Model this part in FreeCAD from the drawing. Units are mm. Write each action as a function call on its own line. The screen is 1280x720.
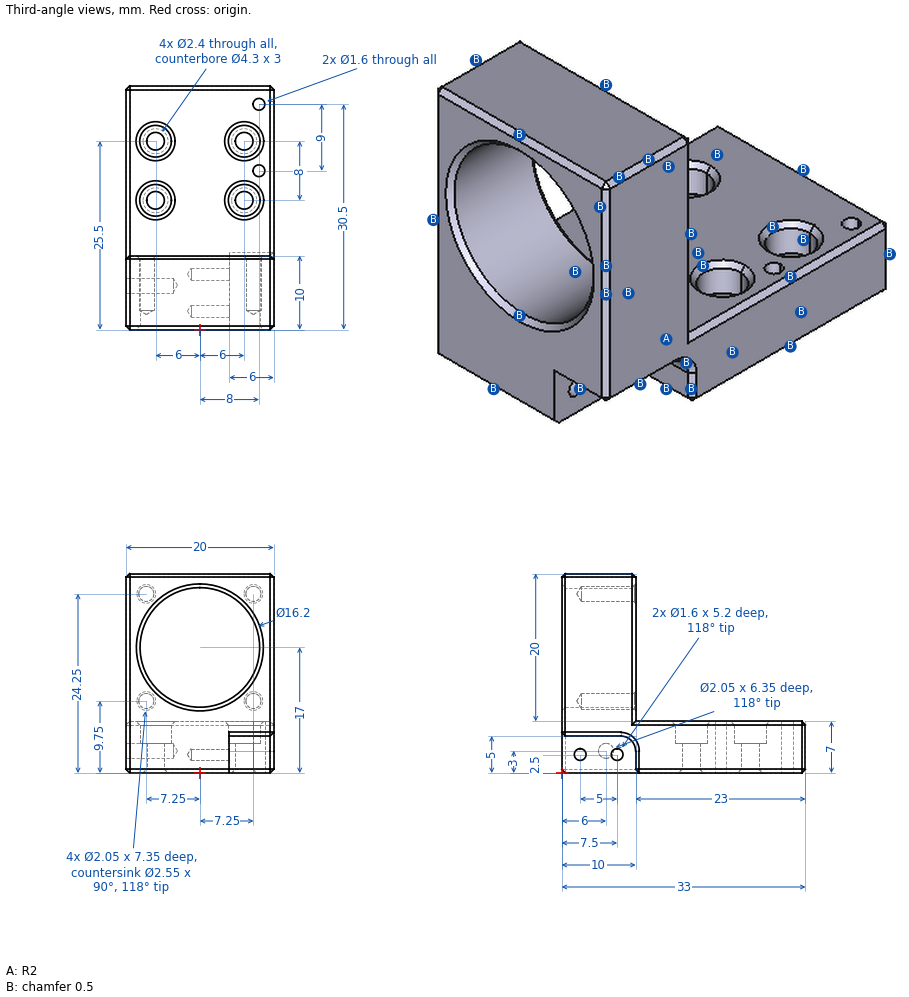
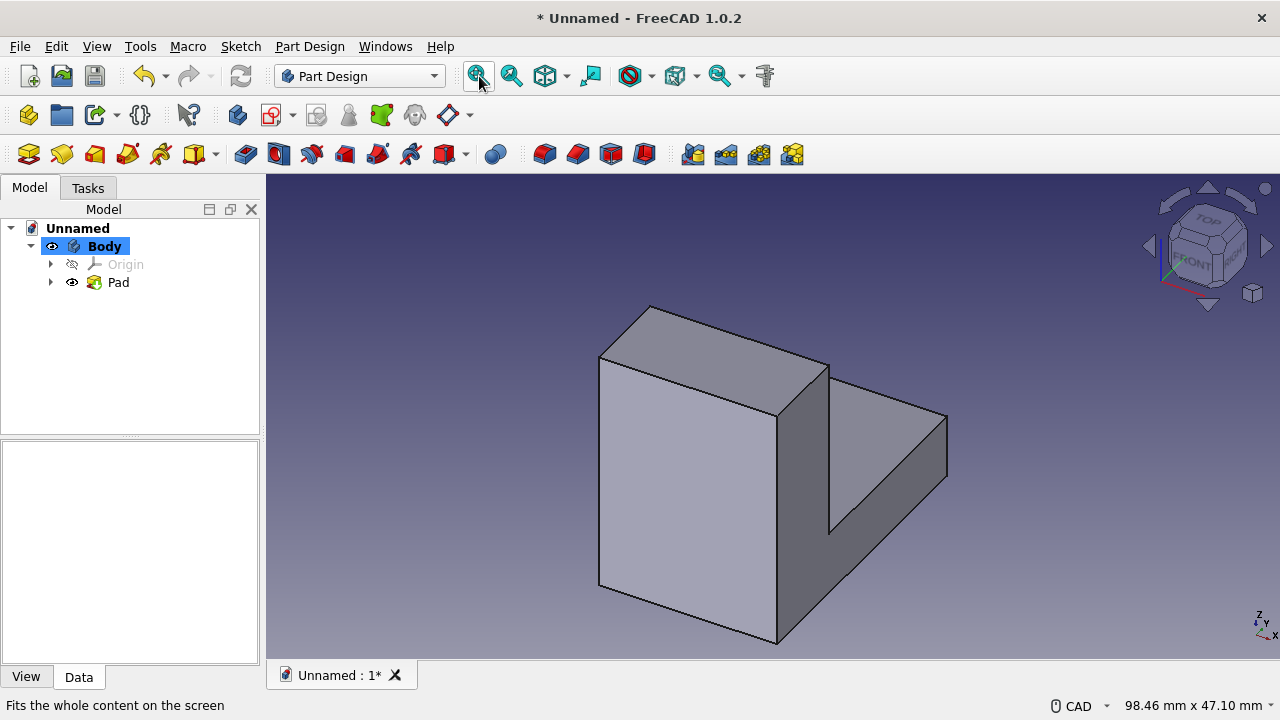
key(4)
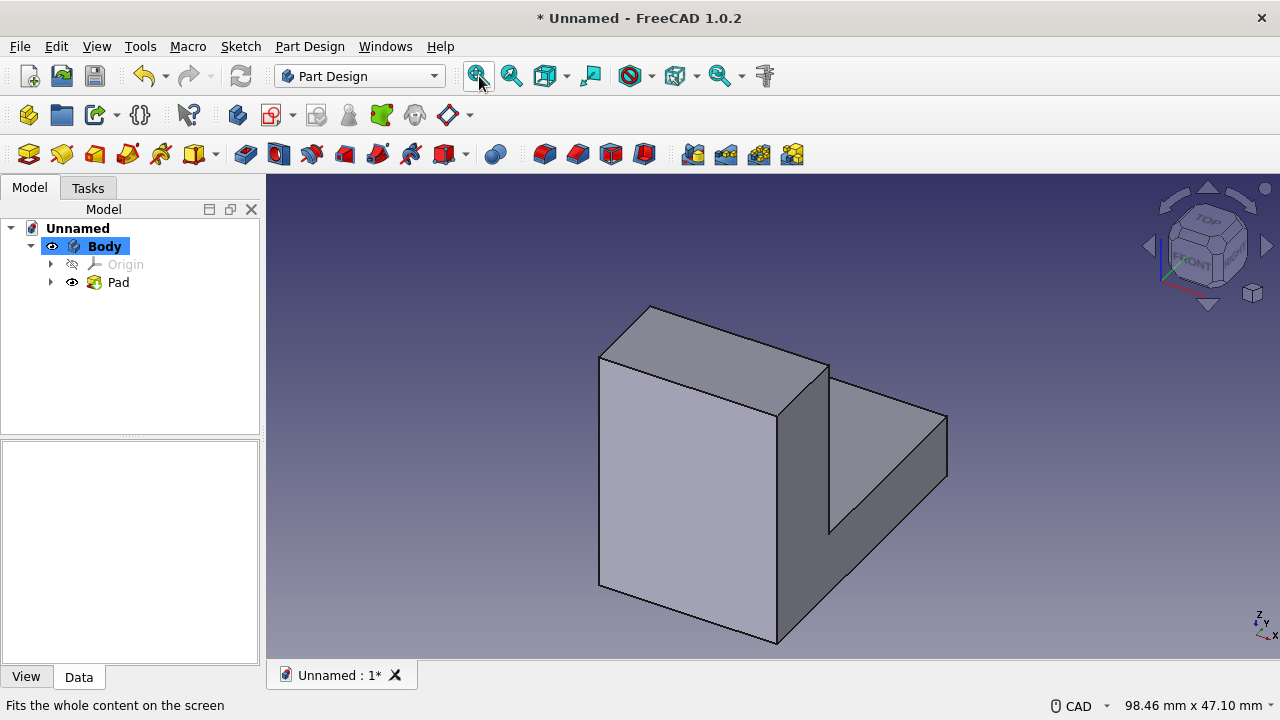
click(773, 379)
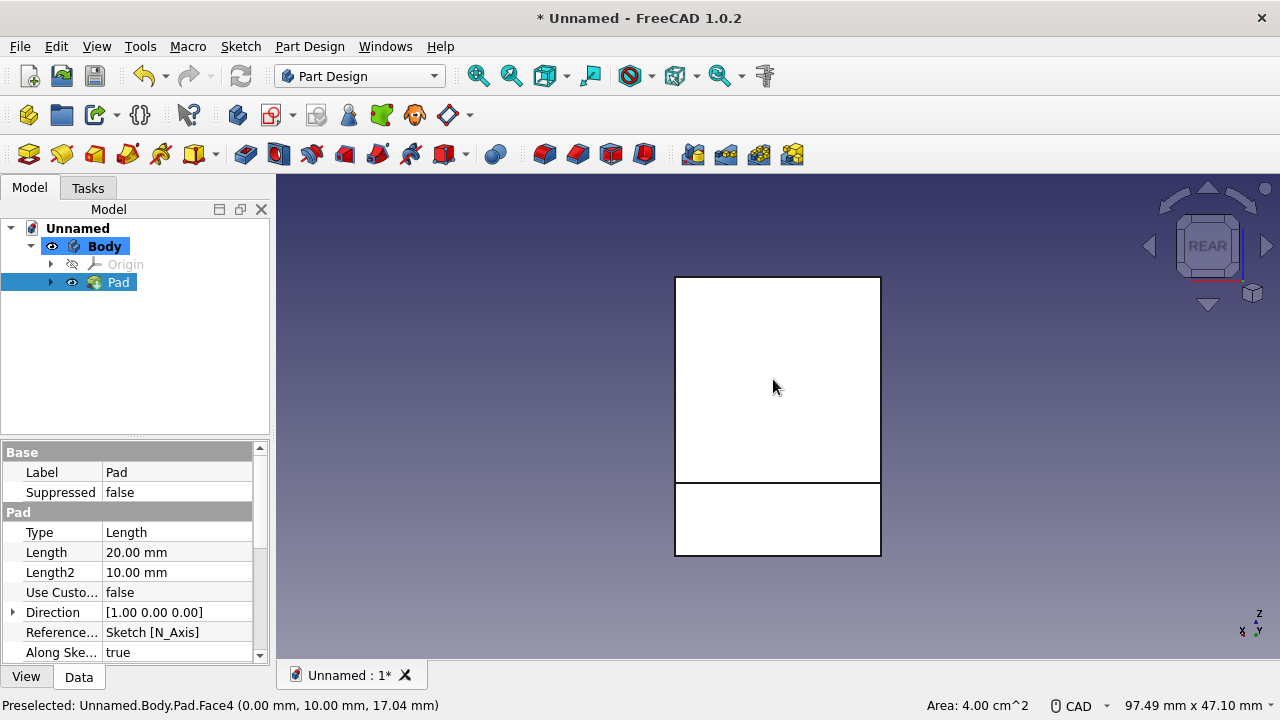
click(270, 116)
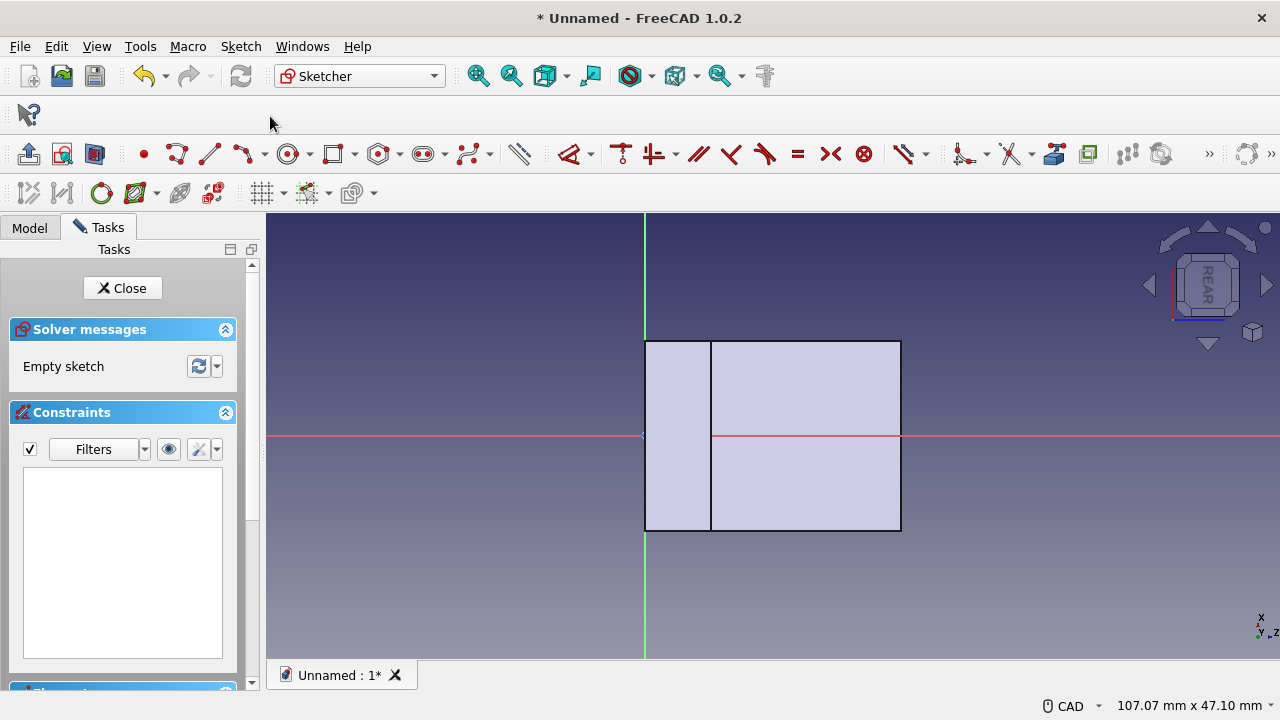
click(95, 154)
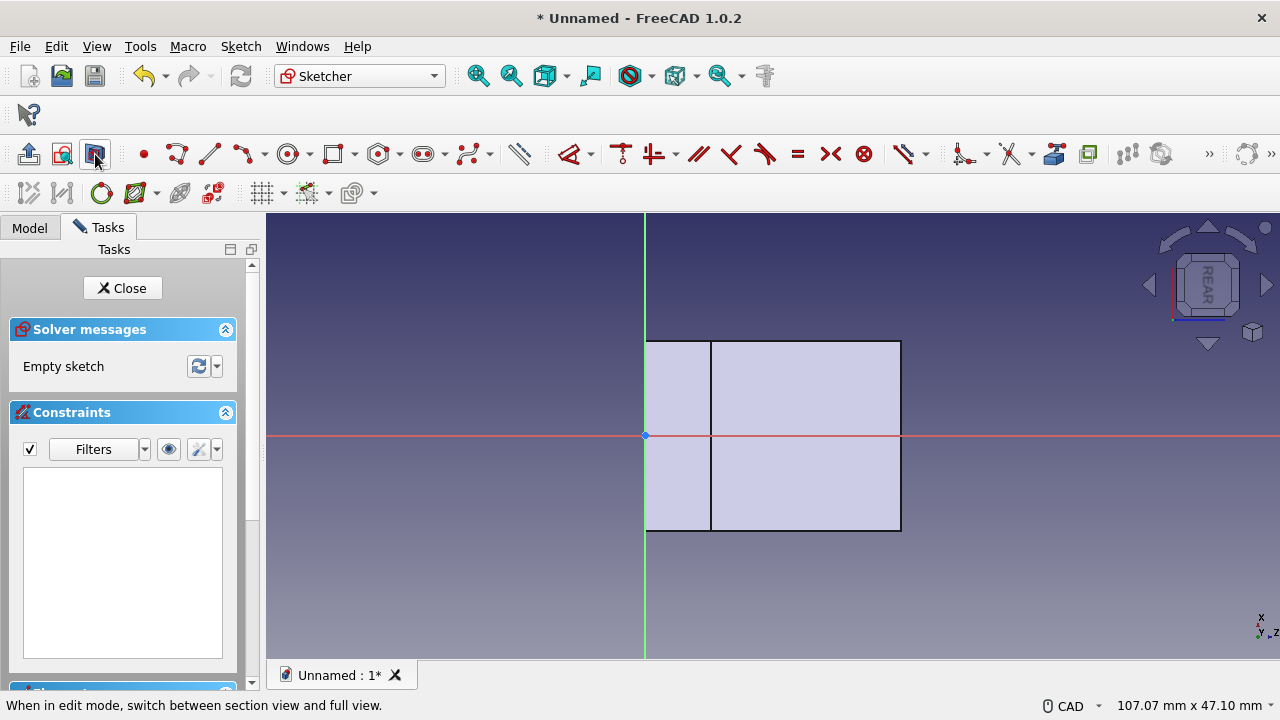
scroll(836, 436, up, 3)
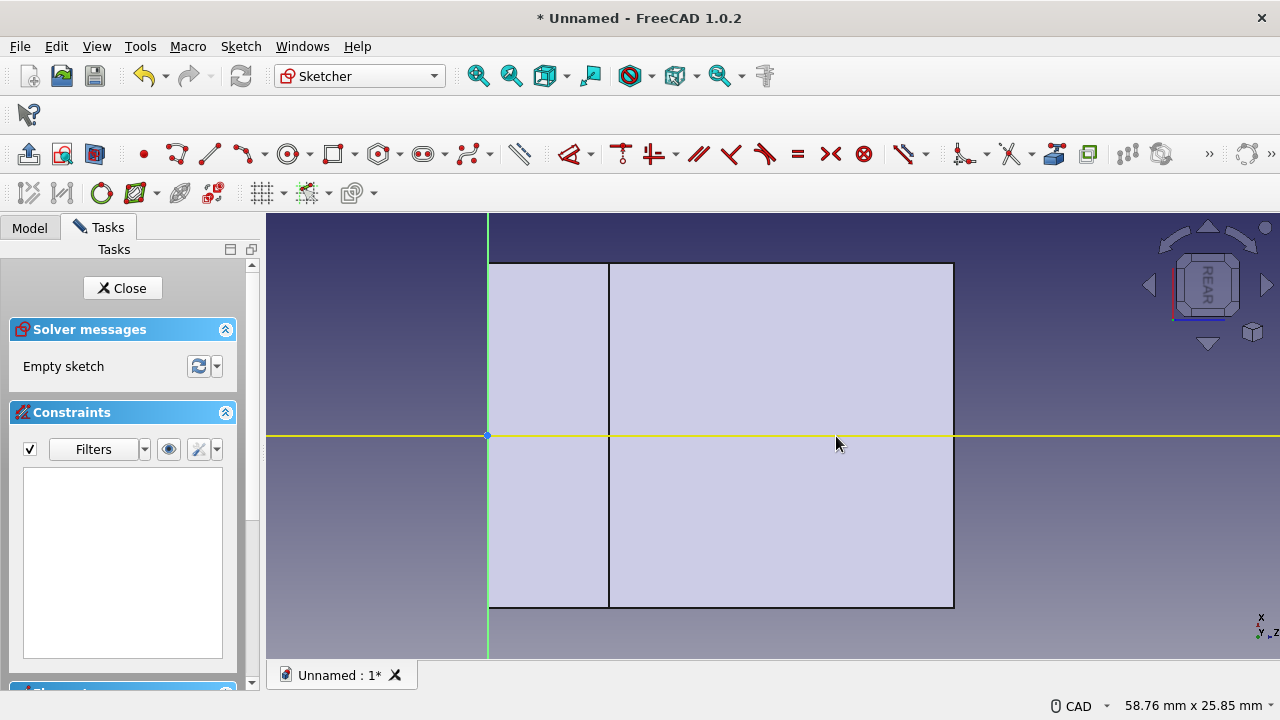
key(g)
key(c)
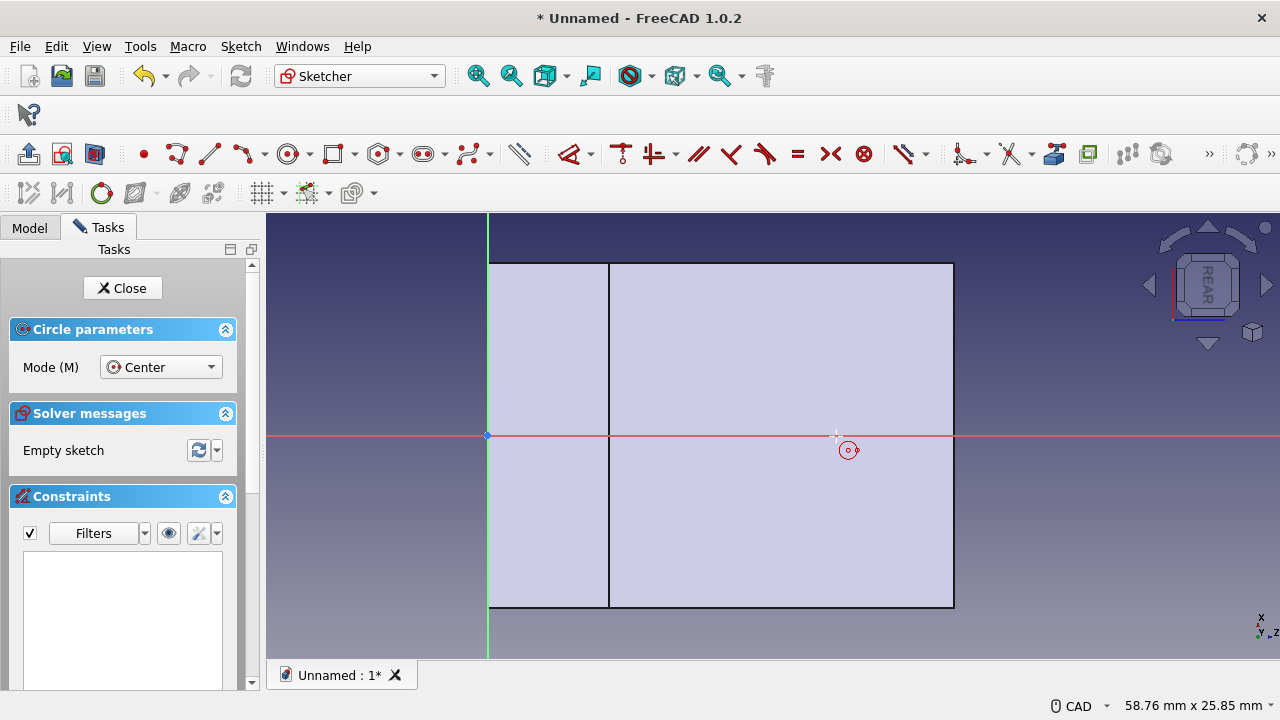
click(781, 436)
move(880, 337)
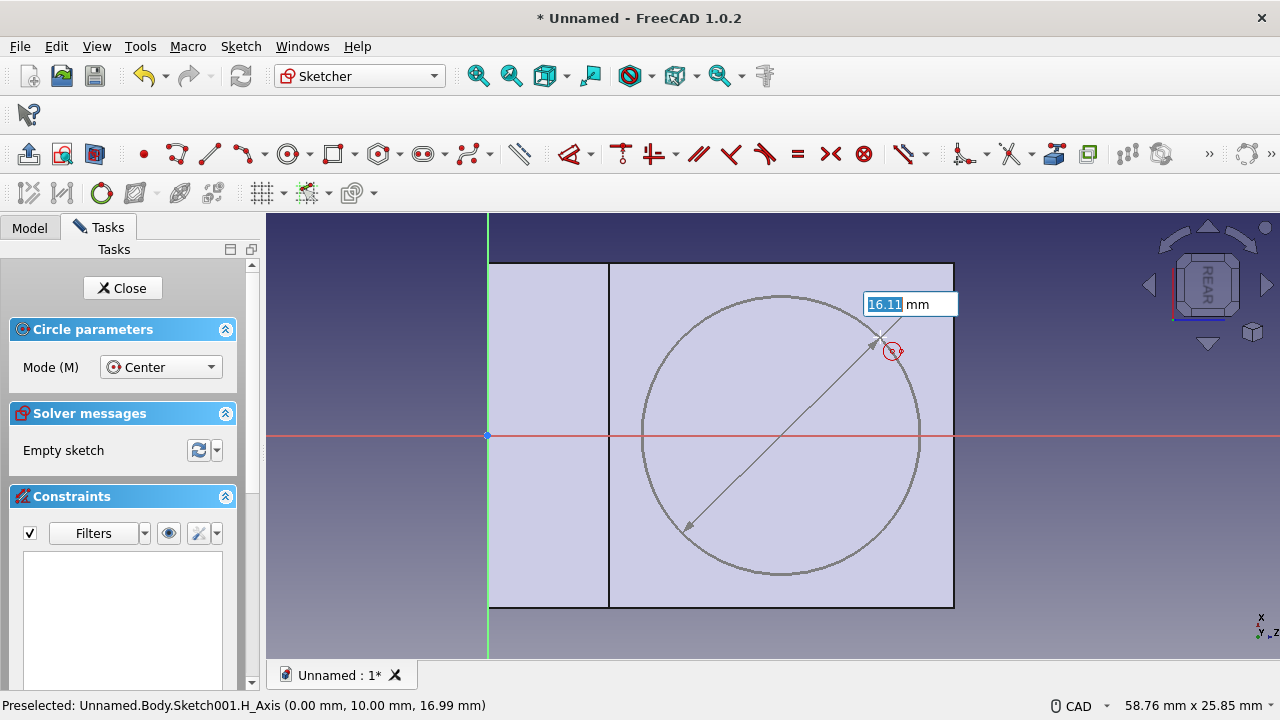
text(16.2)
key(Return)
key(Escape)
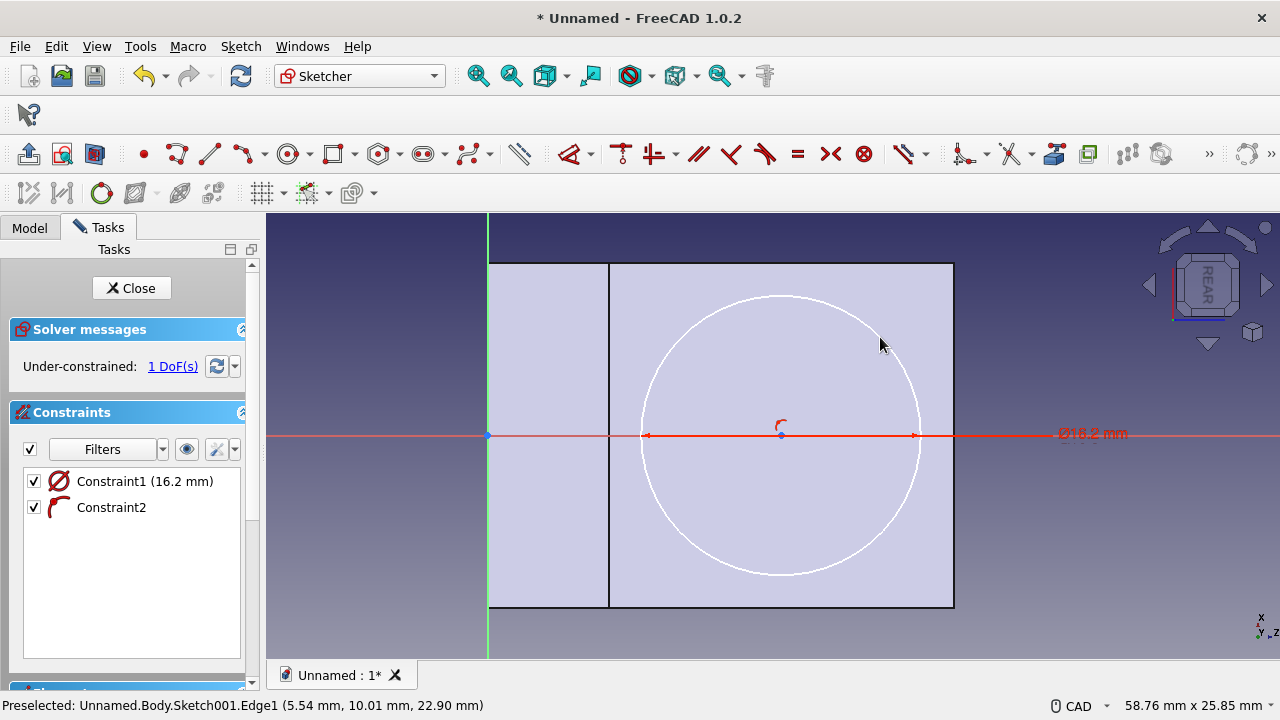
click(568, 154)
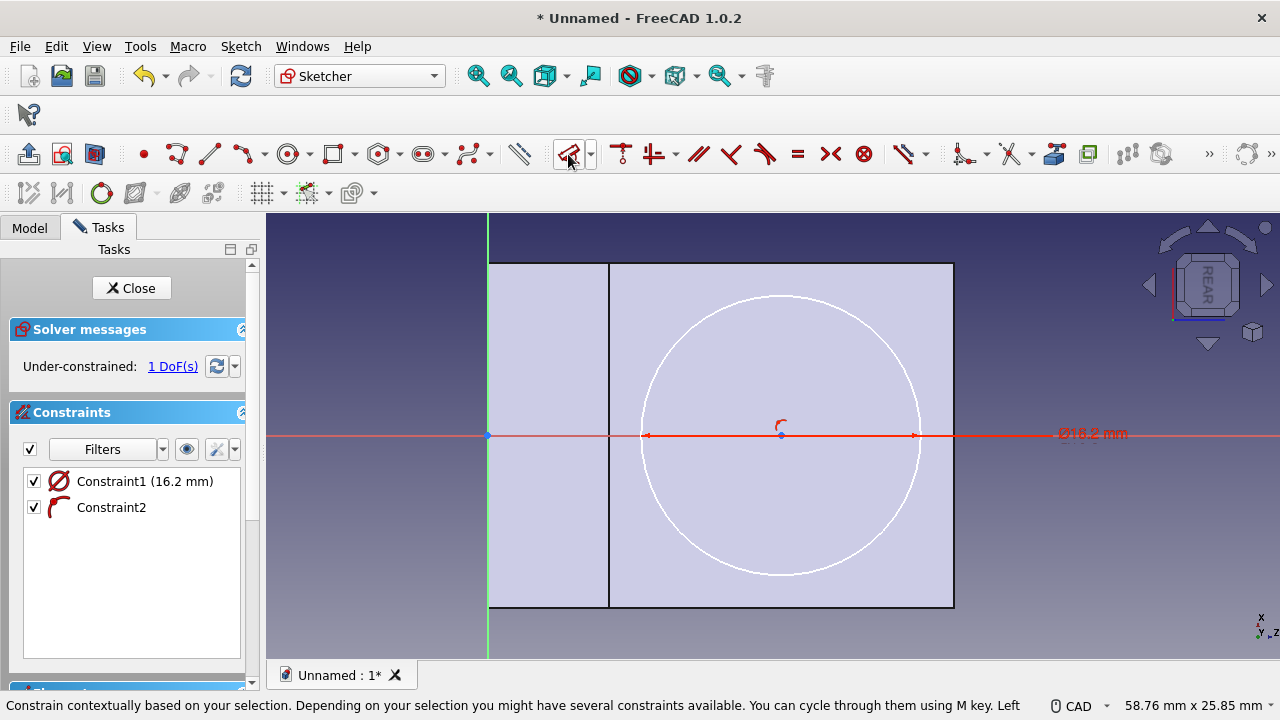
click(781, 436)
click(567, 470)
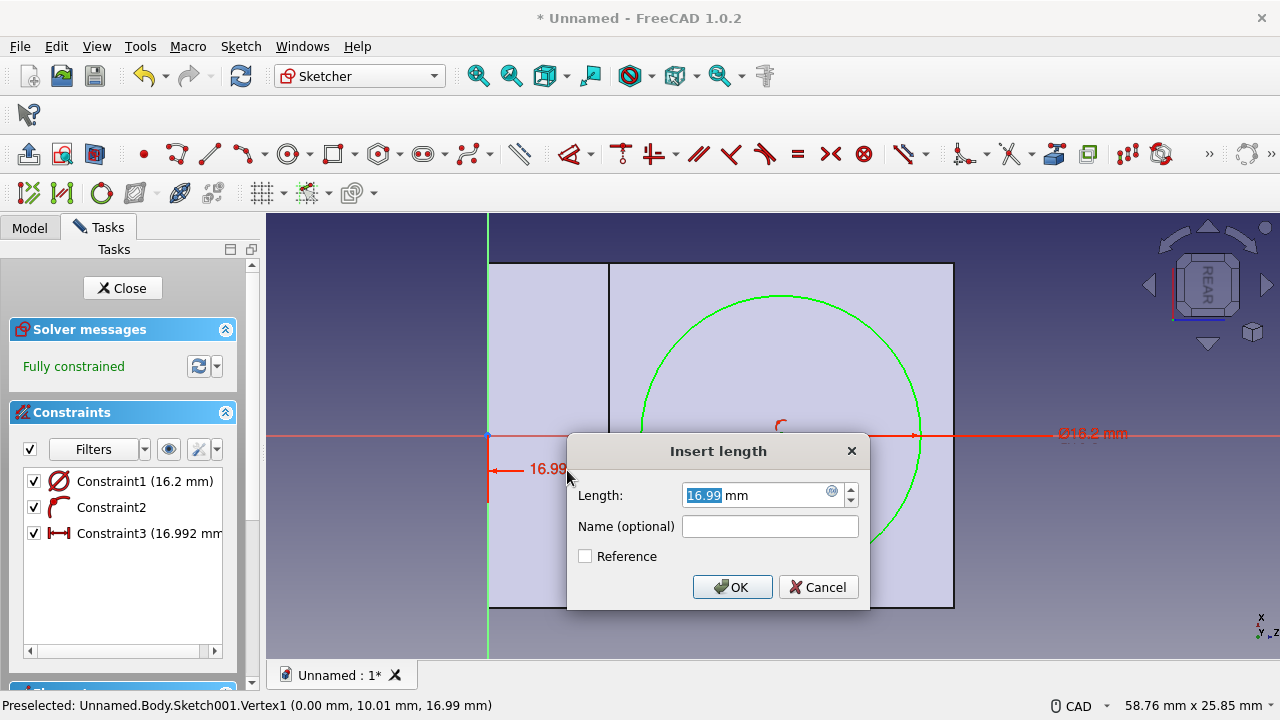
text(17)
key(Return)
key(Escape)